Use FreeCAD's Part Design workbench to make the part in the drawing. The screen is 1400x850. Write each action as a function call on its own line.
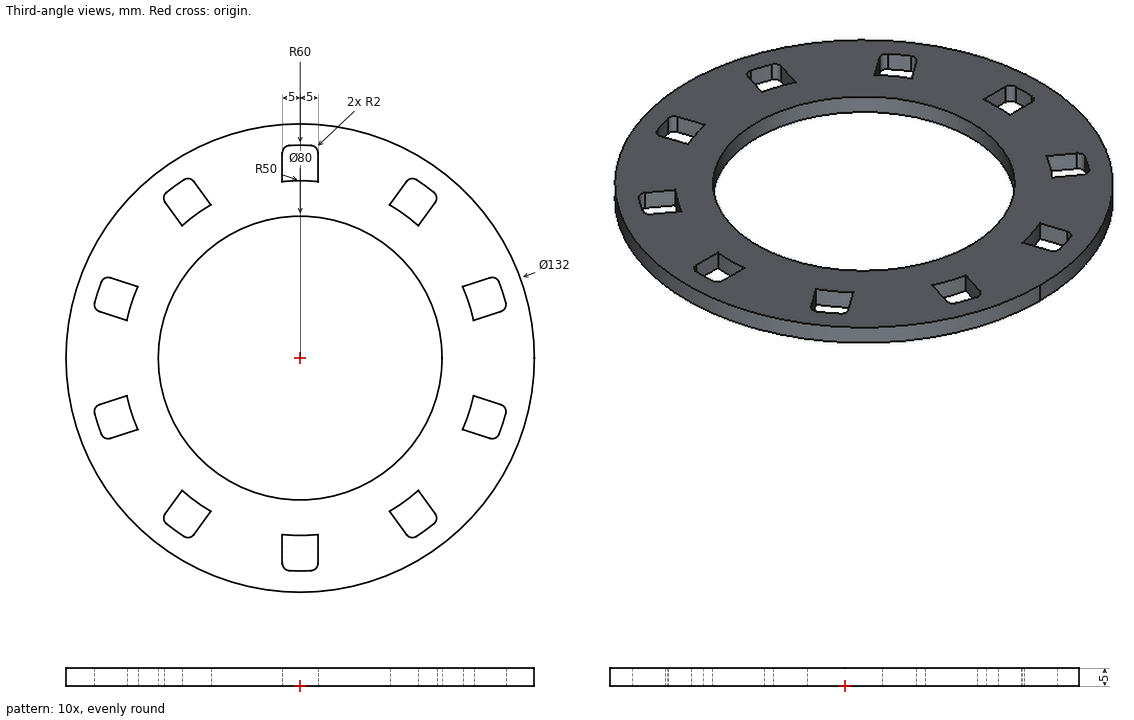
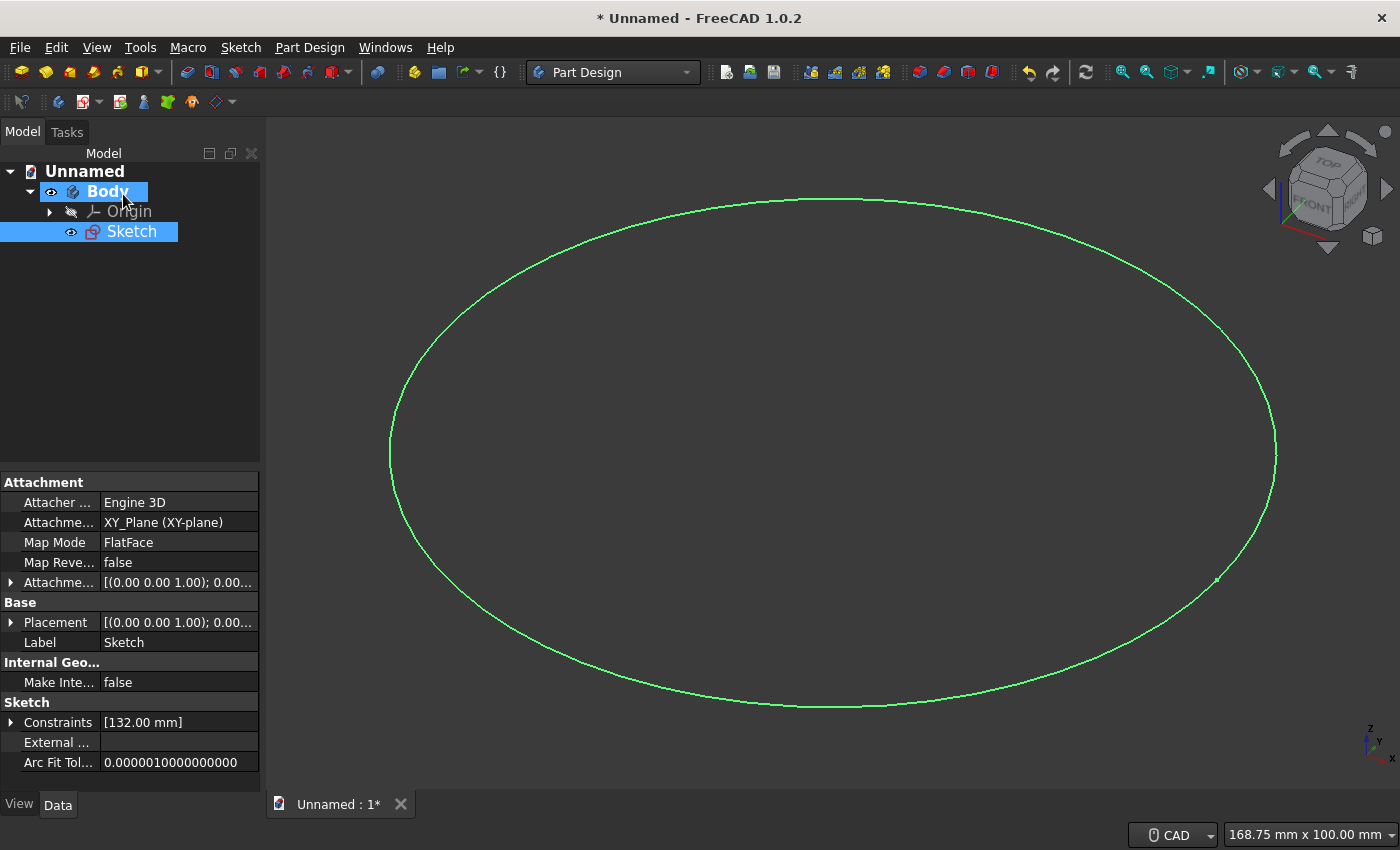
click(22, 72)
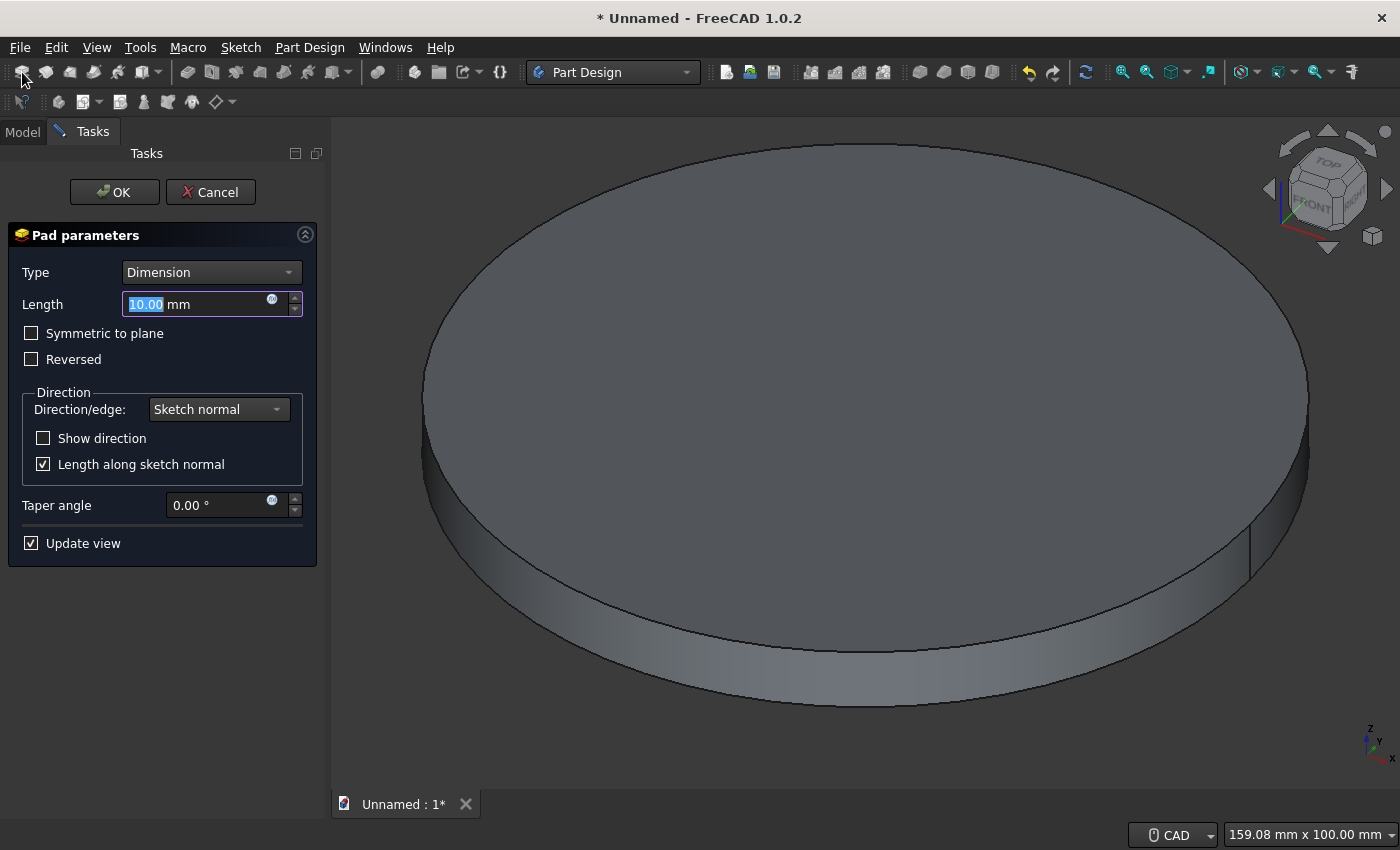
text(5)
key(Tab)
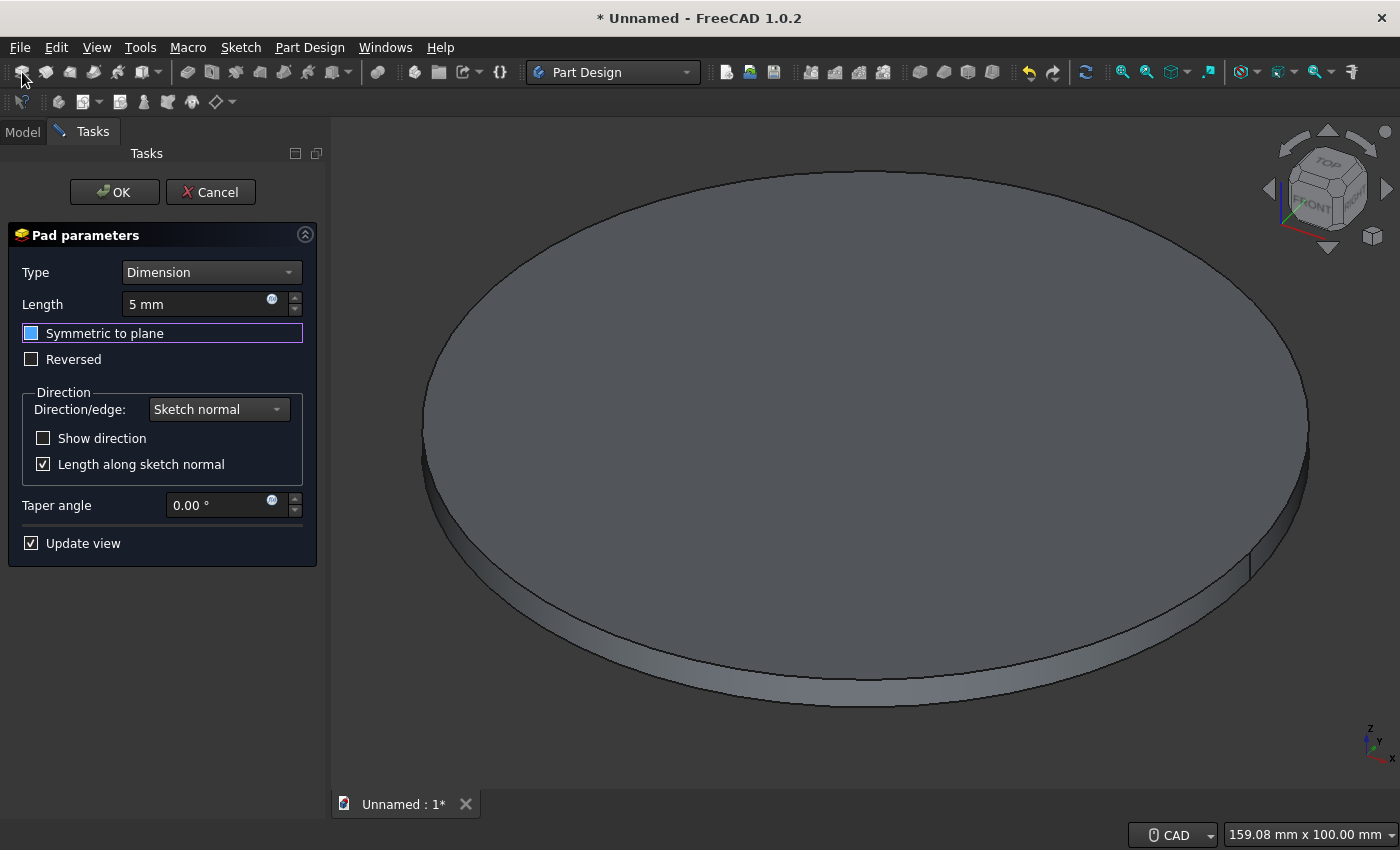
click(115, 192)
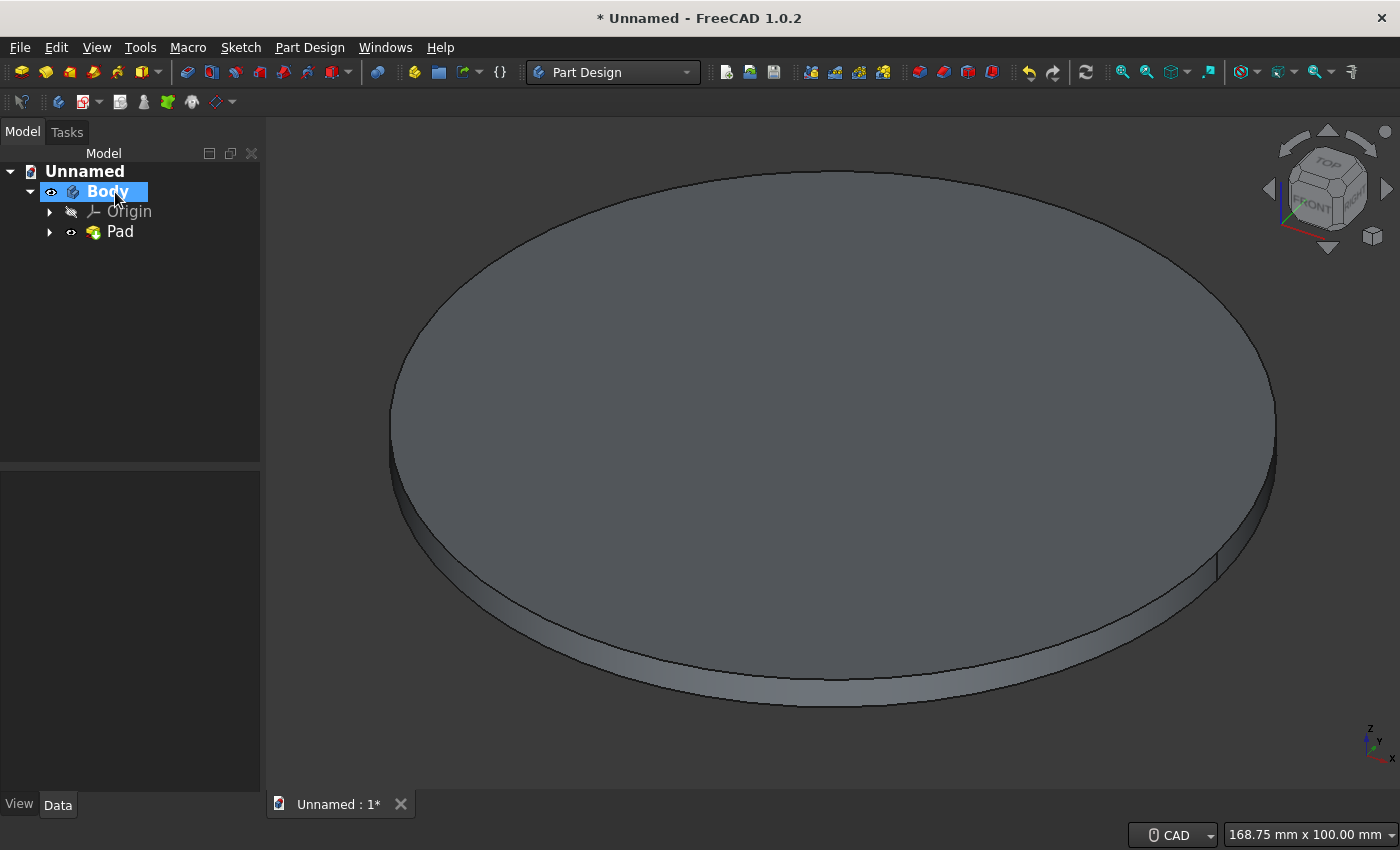
click(1124, 72)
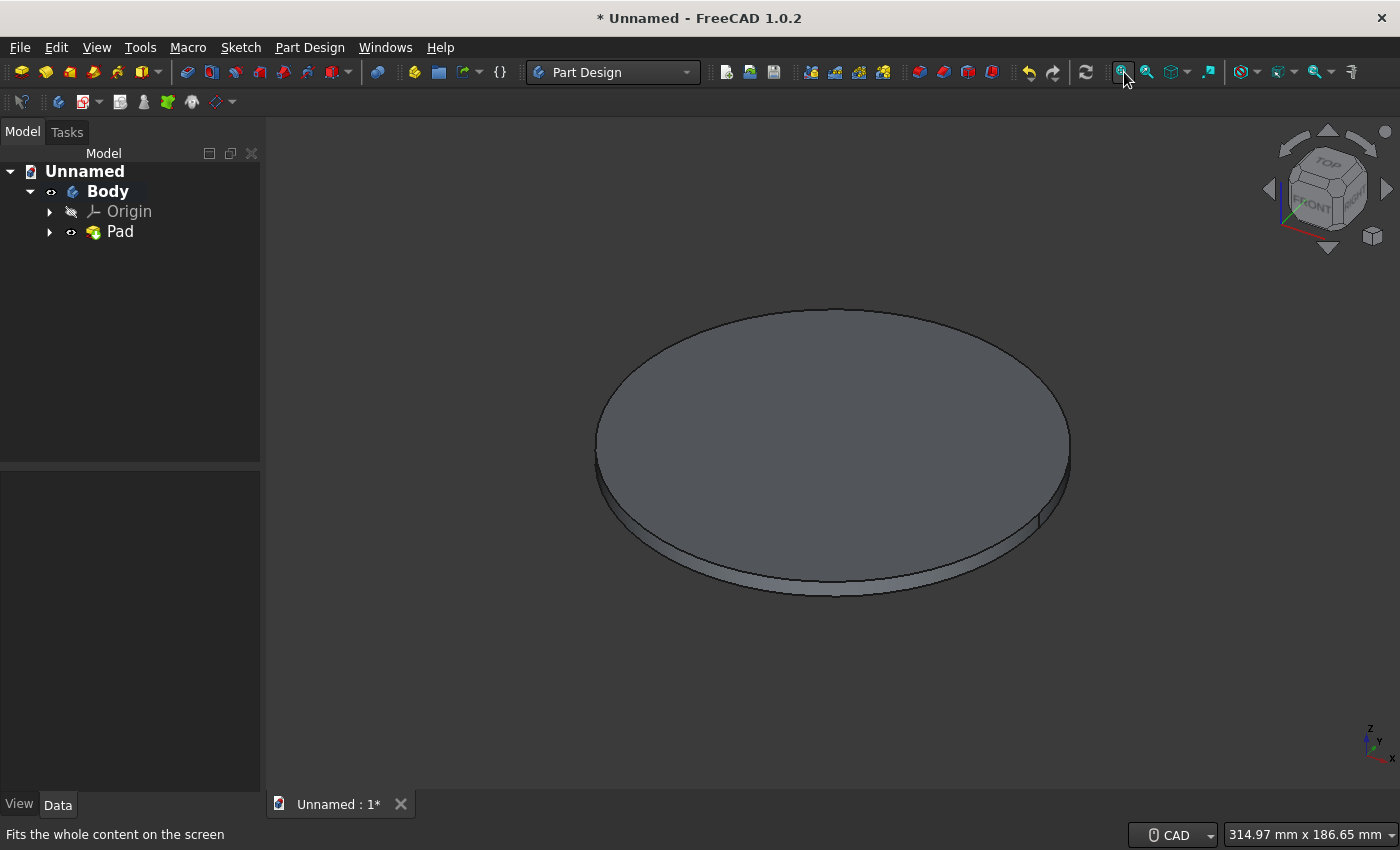
click(833, 445)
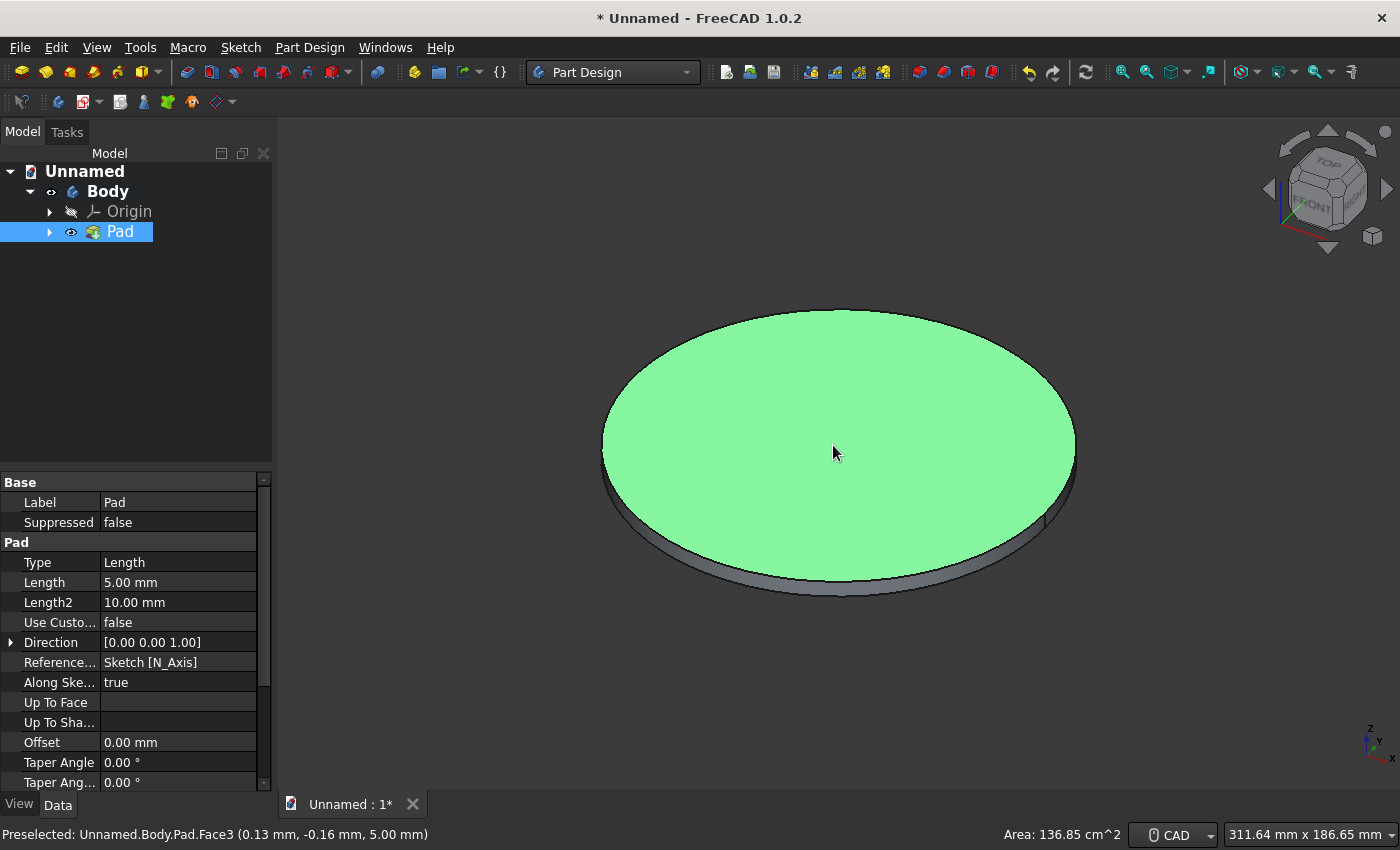
click(84, 102)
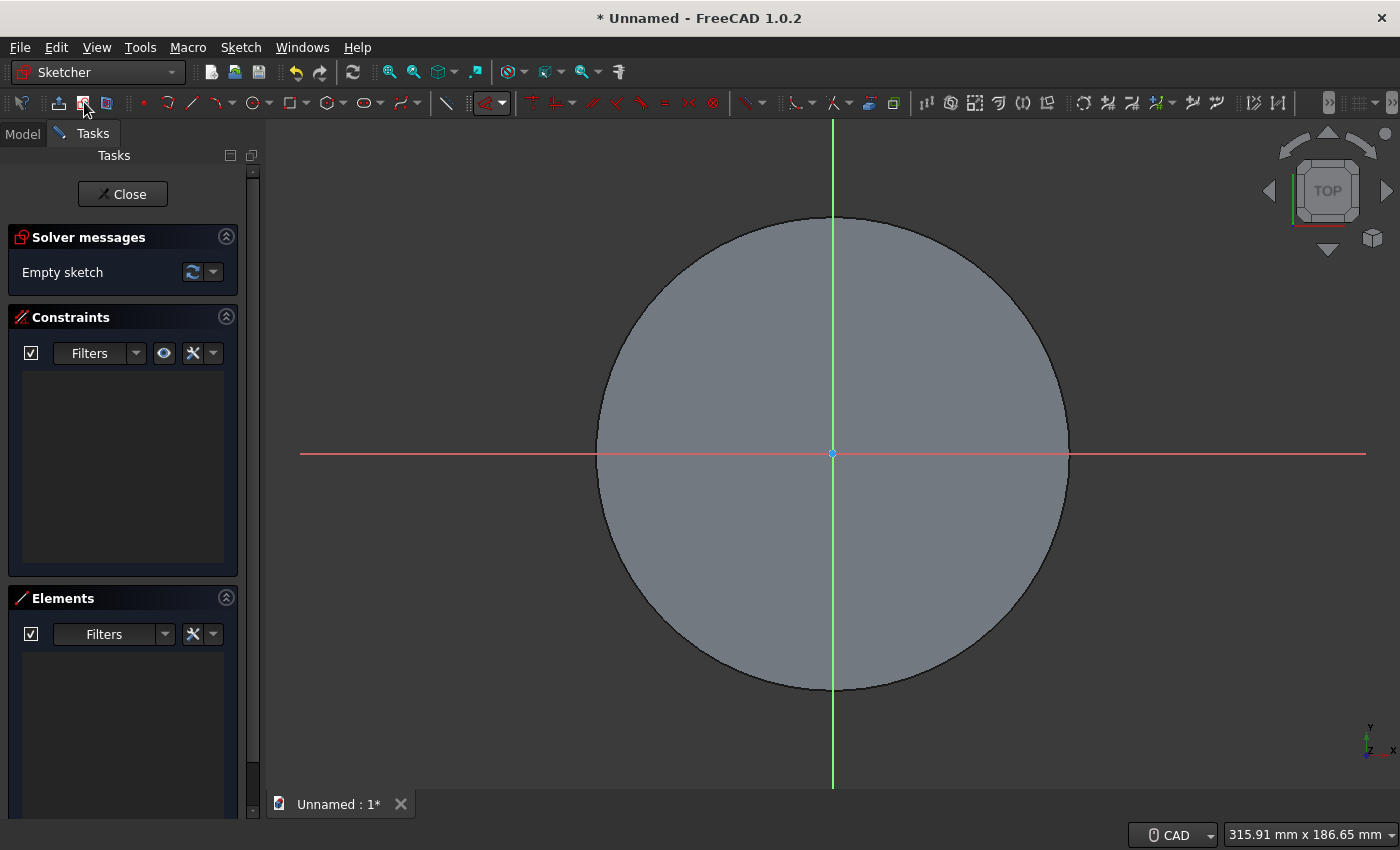
scroll(840, 237, up, 12)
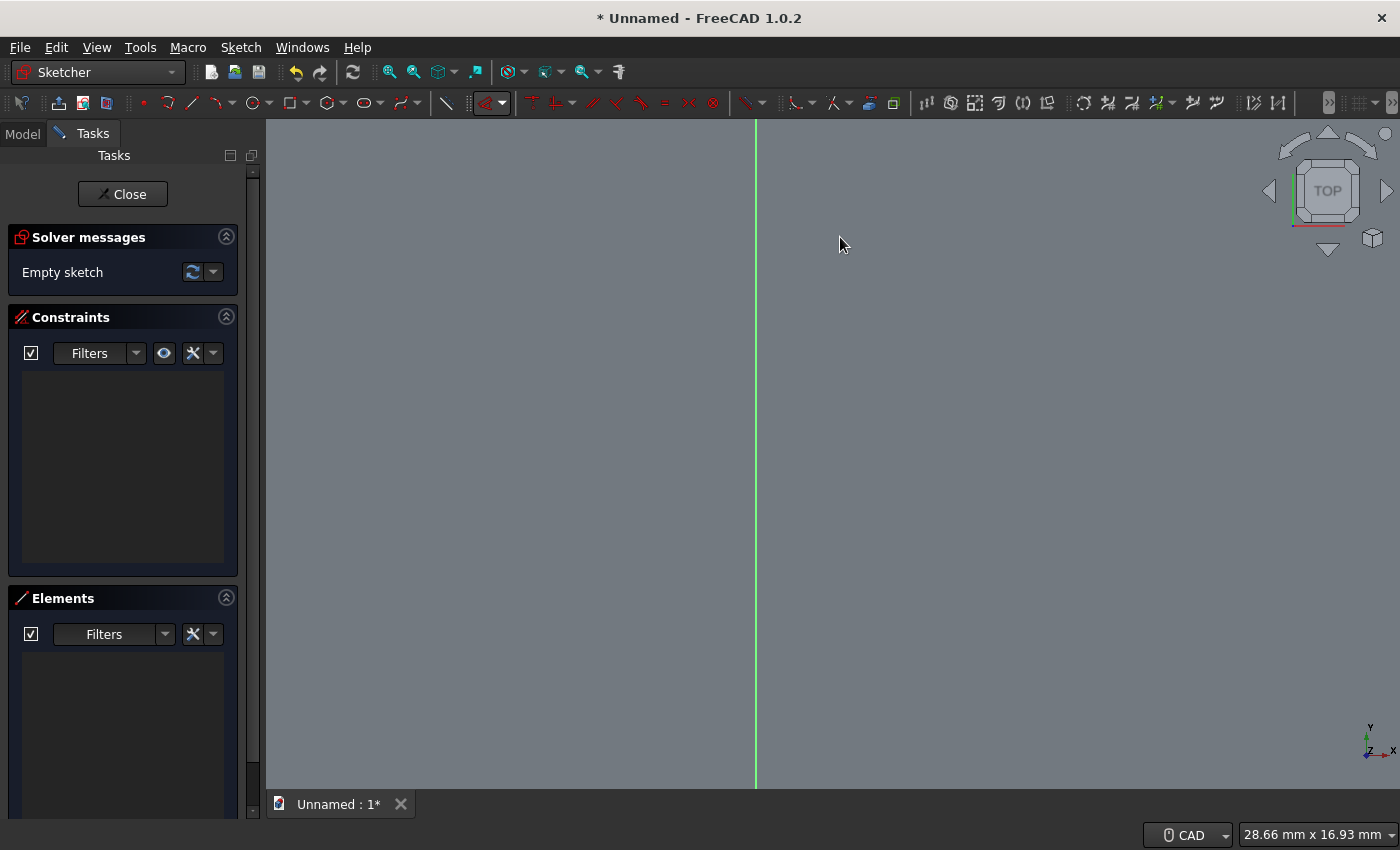
key(g)
key(l)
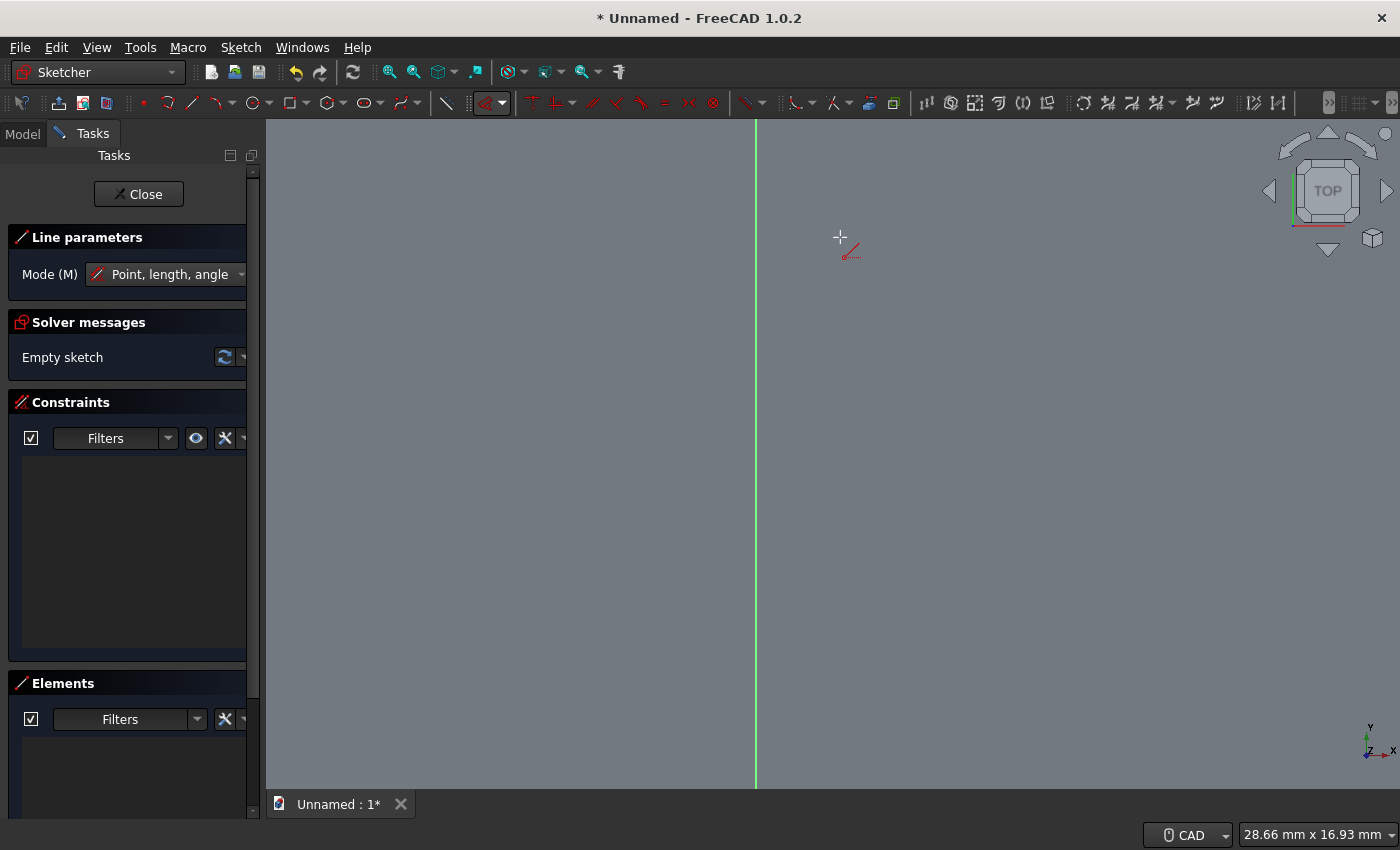
click(954, 659)
click(954, 335)